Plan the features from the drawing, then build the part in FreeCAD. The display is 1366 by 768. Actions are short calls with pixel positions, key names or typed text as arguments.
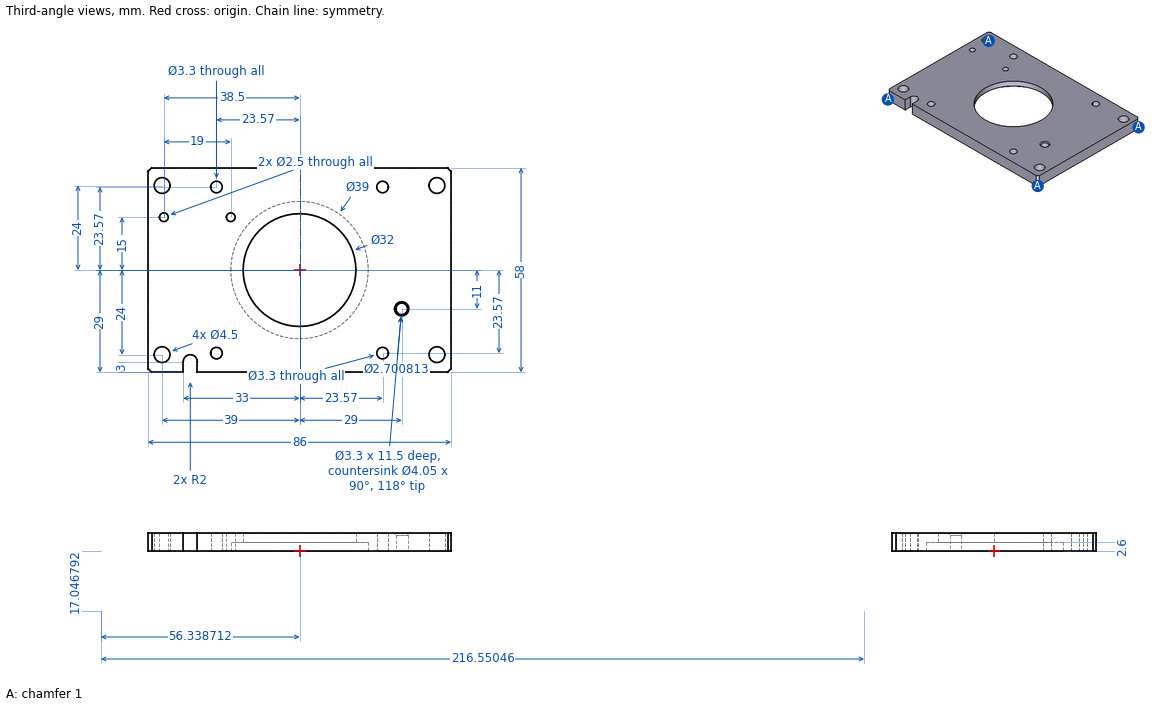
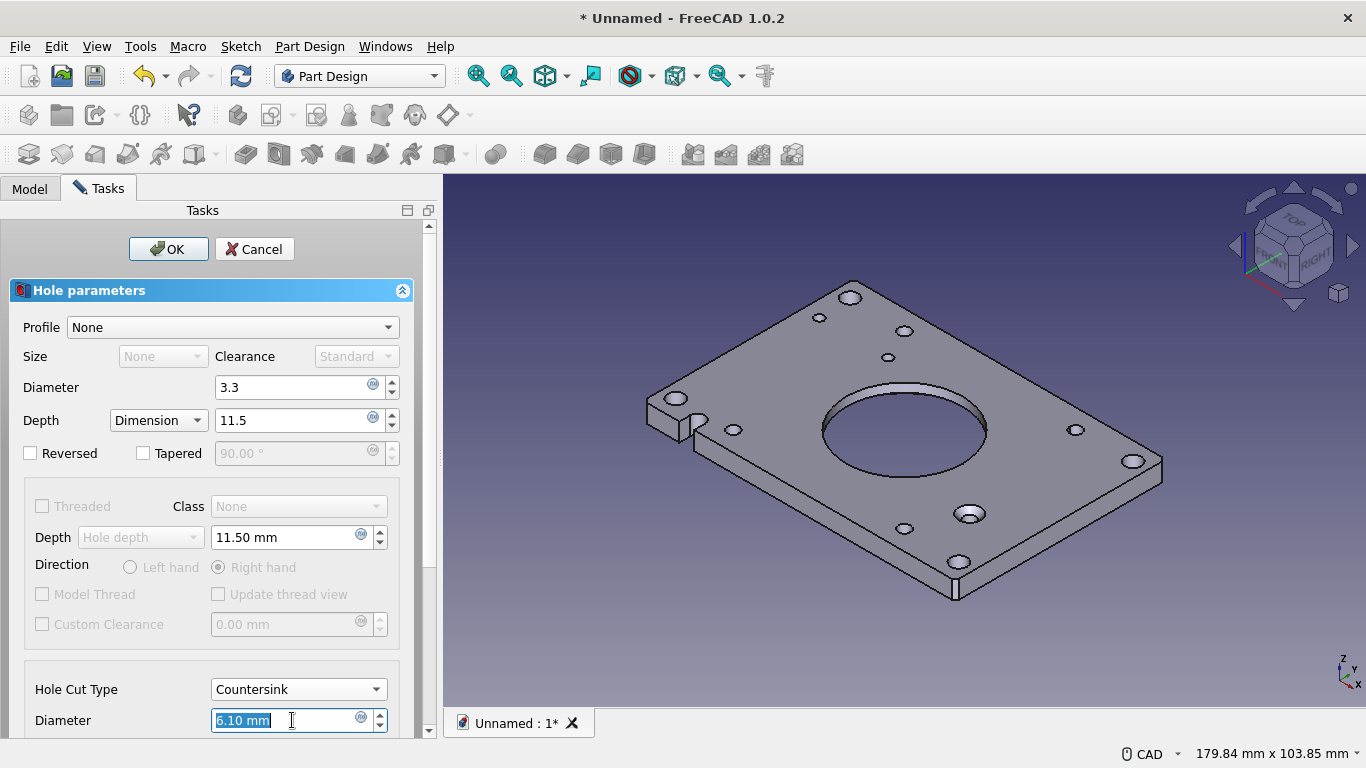
text(4.05)
key(Tab)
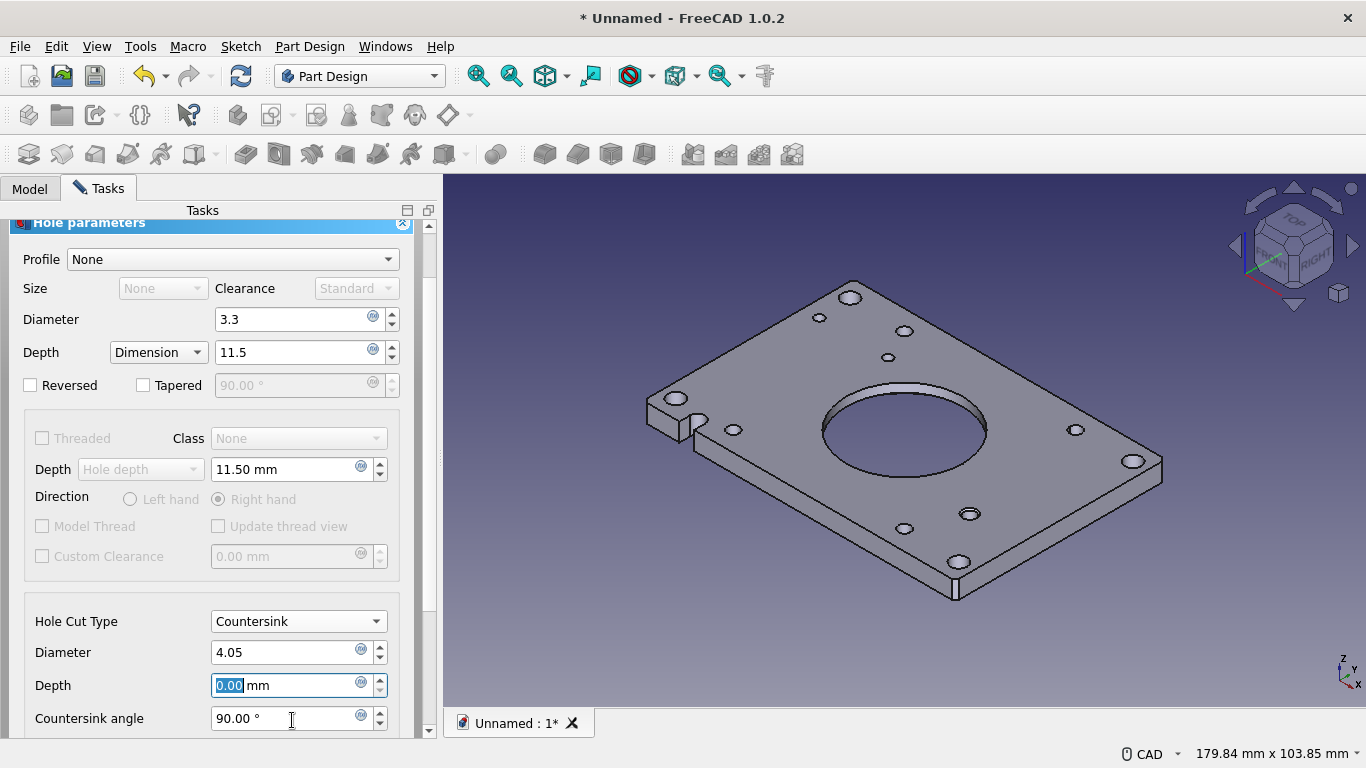
scroll(429, 479, up, 2)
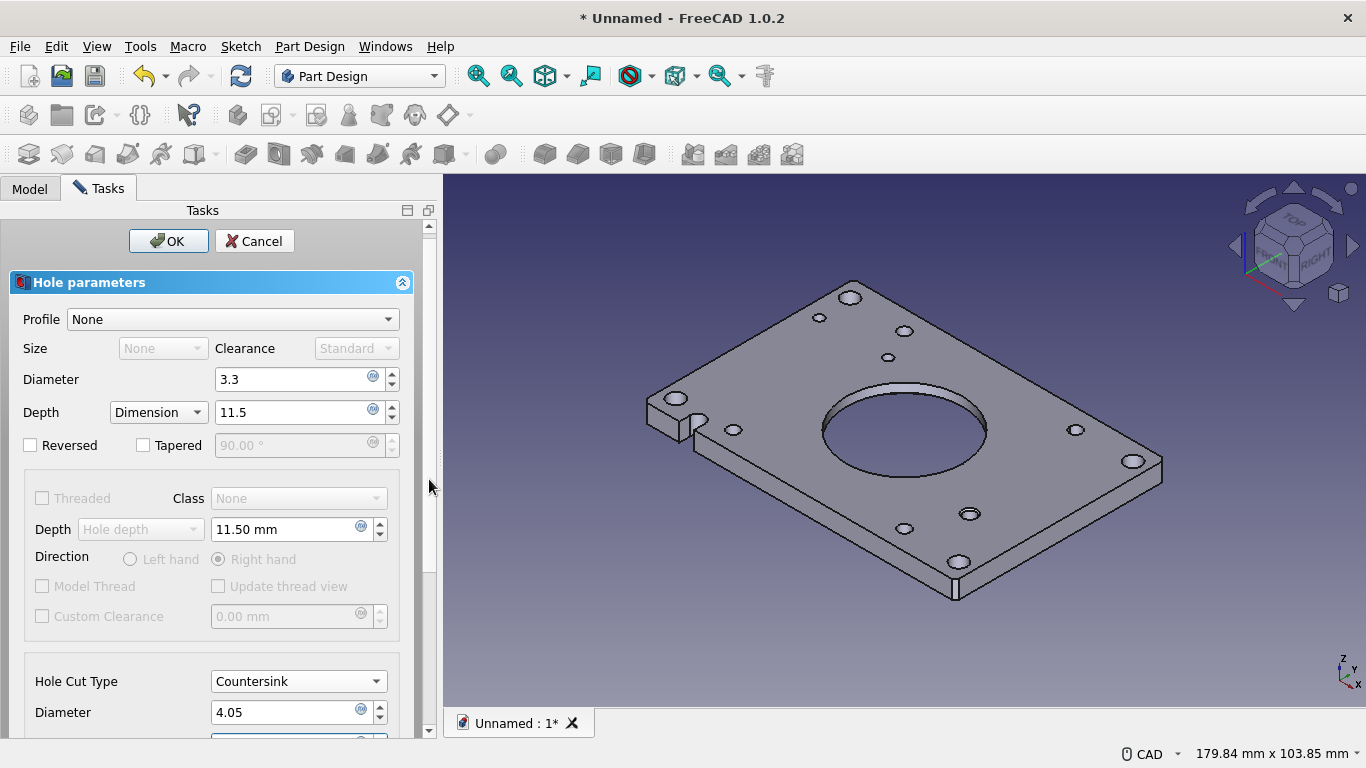
click(169, 249)